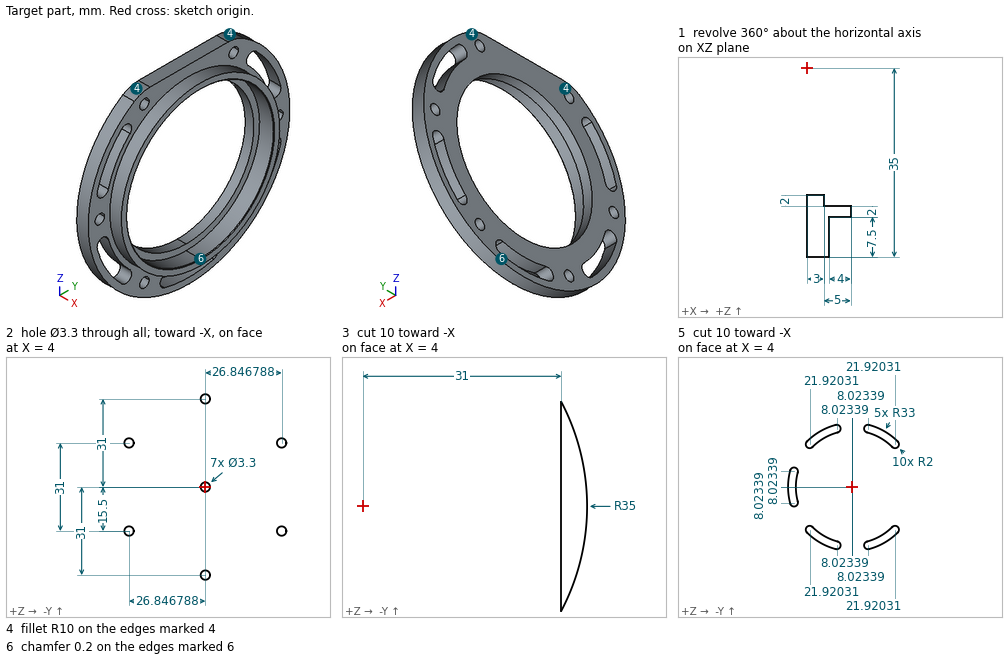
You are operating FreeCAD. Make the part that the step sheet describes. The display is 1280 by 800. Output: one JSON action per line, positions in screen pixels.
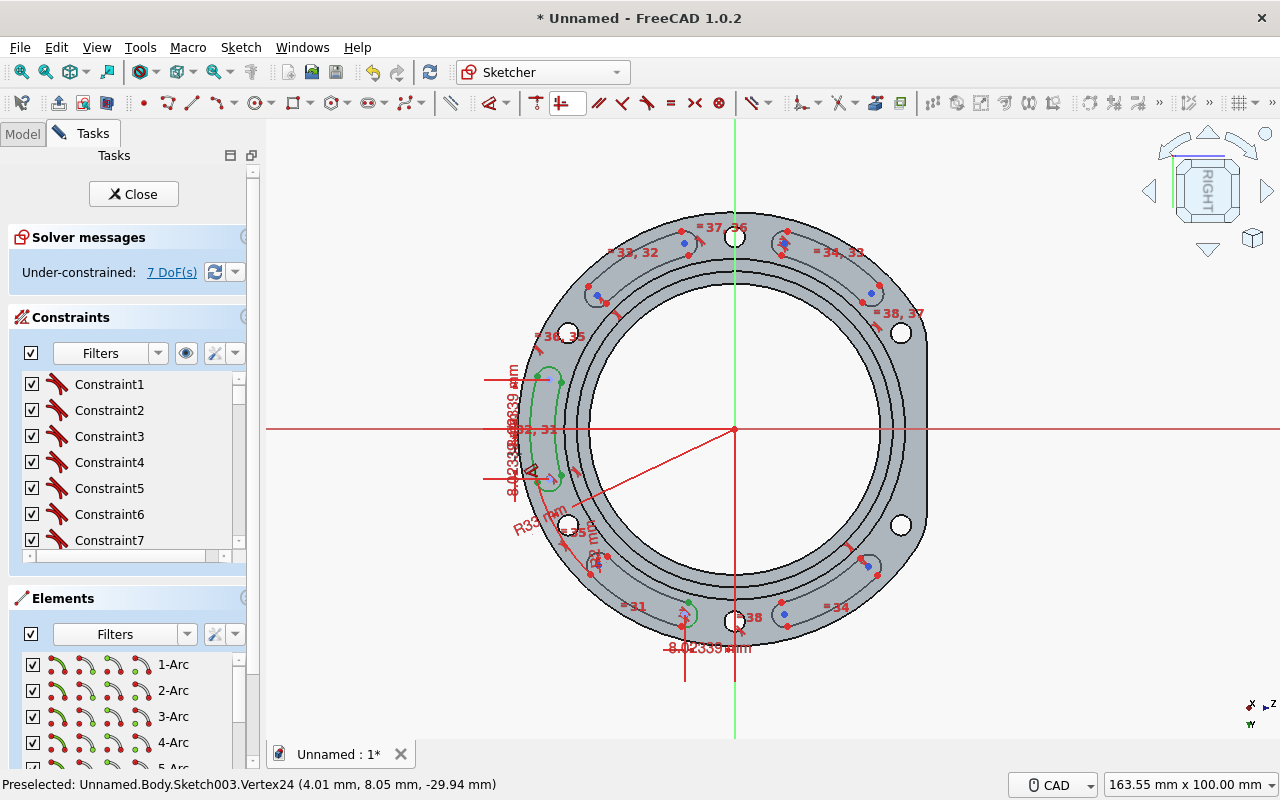
{"action": "left_click", "coordinate": [685, 244]}
{"action": "left_click", "coordinate": [710, 210]}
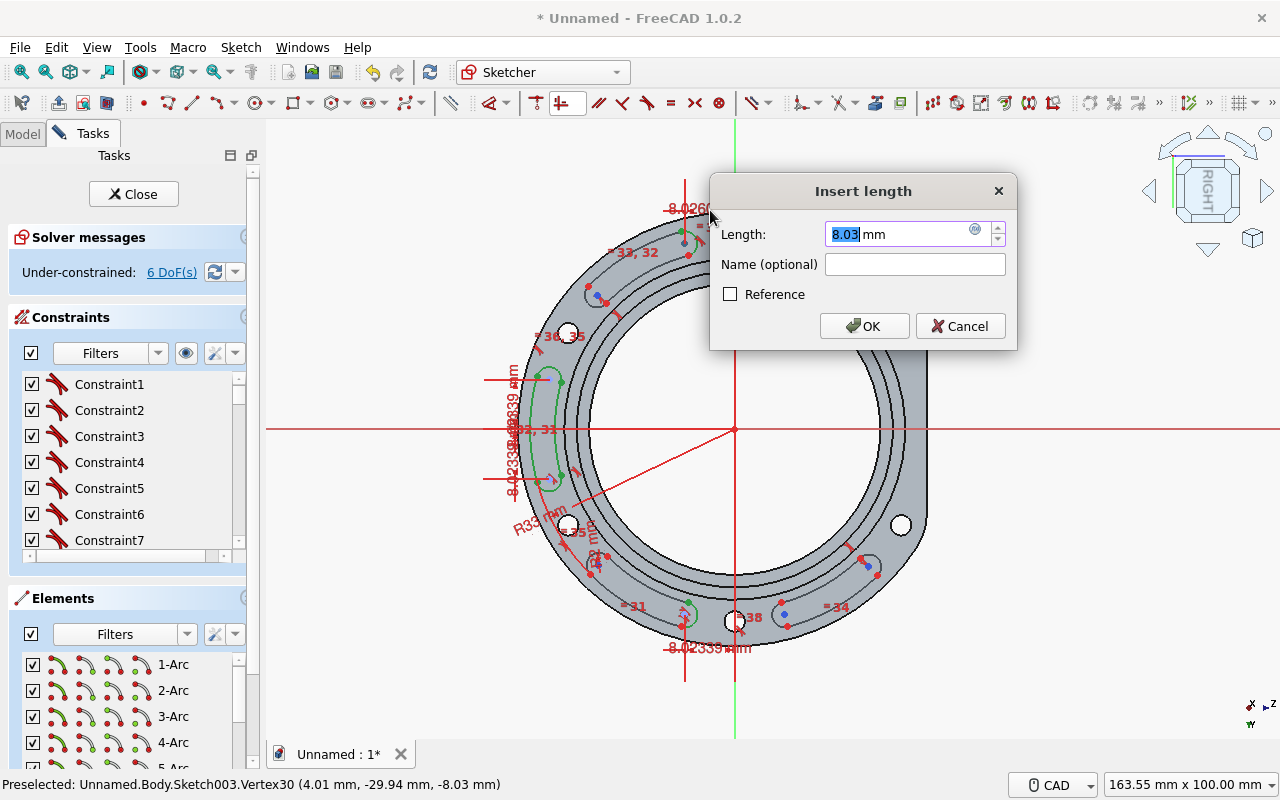
{"action": "type", "text": "8.02339"}
{"action": "key", "text": "Return"}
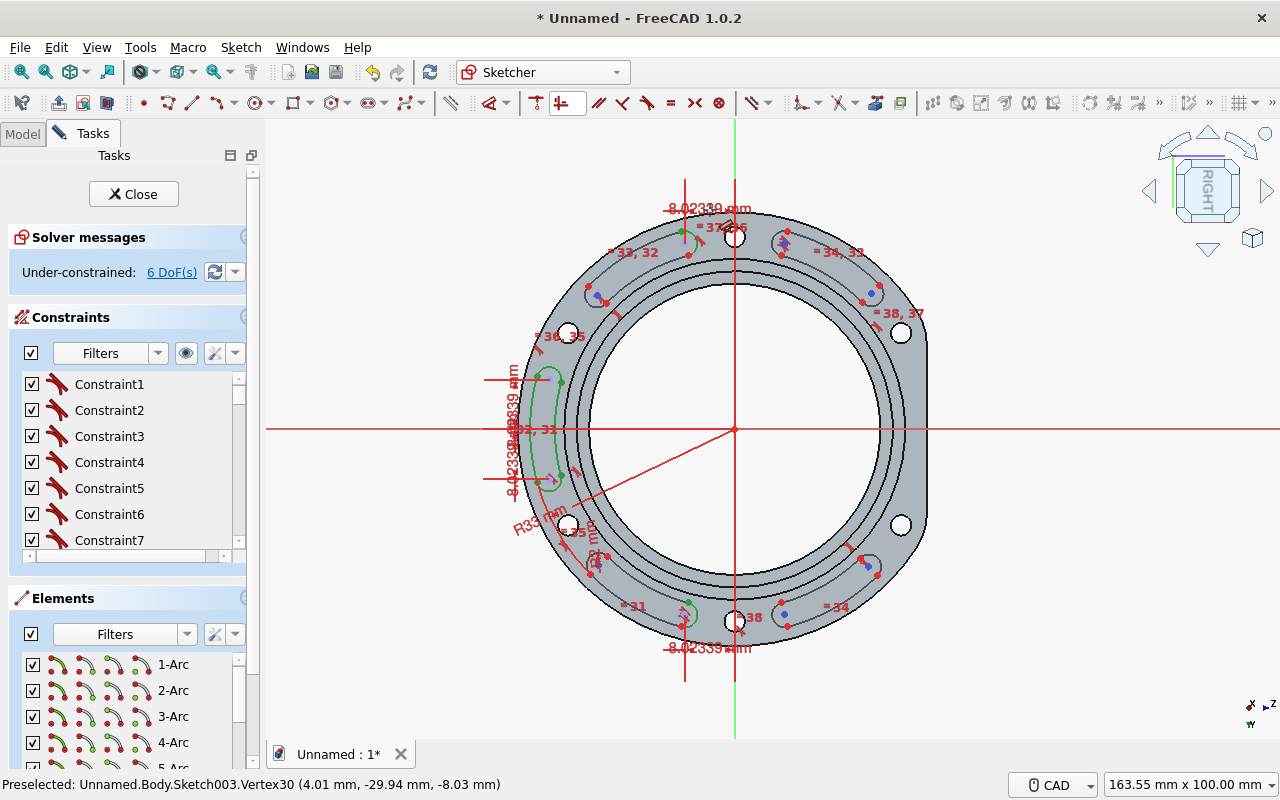
{"action": "left_click", "coordinate": [784, 244]}
{"action": "left_click", "coordinate": [759, 463]}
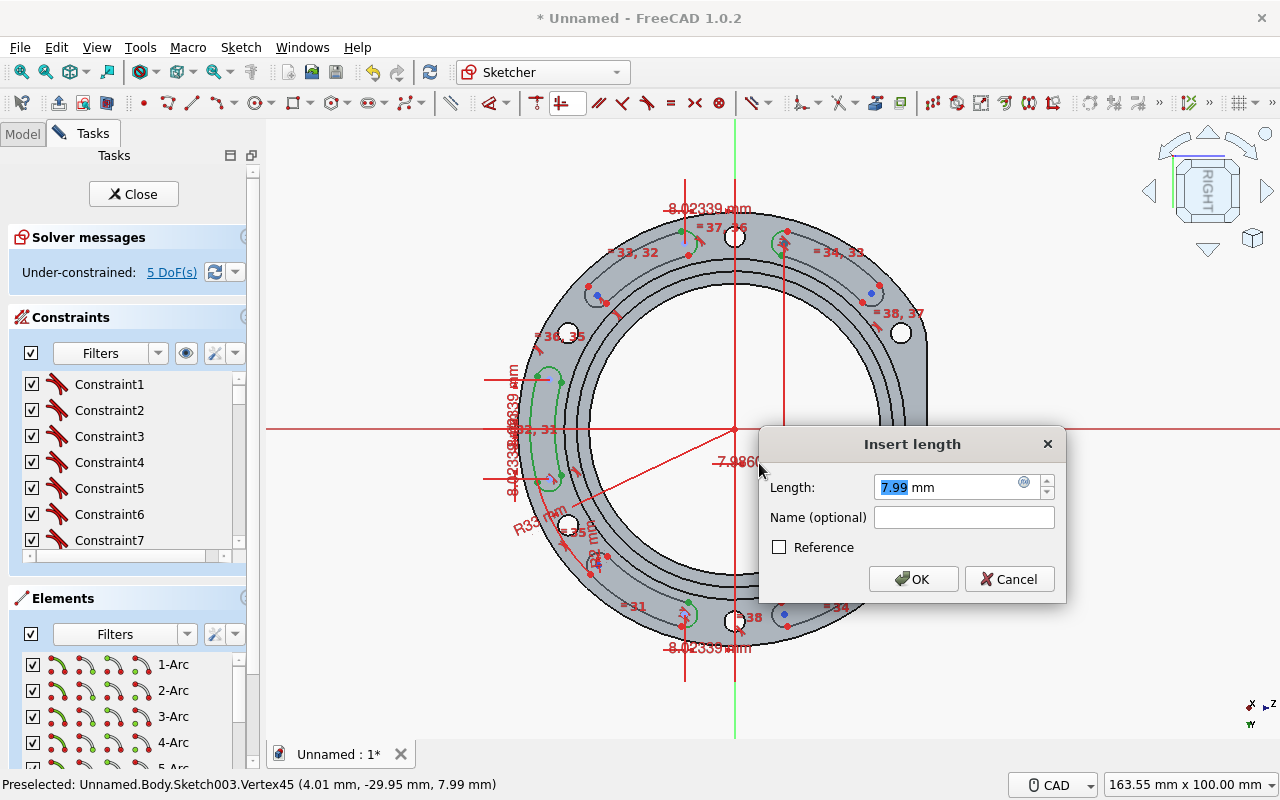
{"action": "type", "text": "8.02339"}
{"action": "key", "text": "Return"}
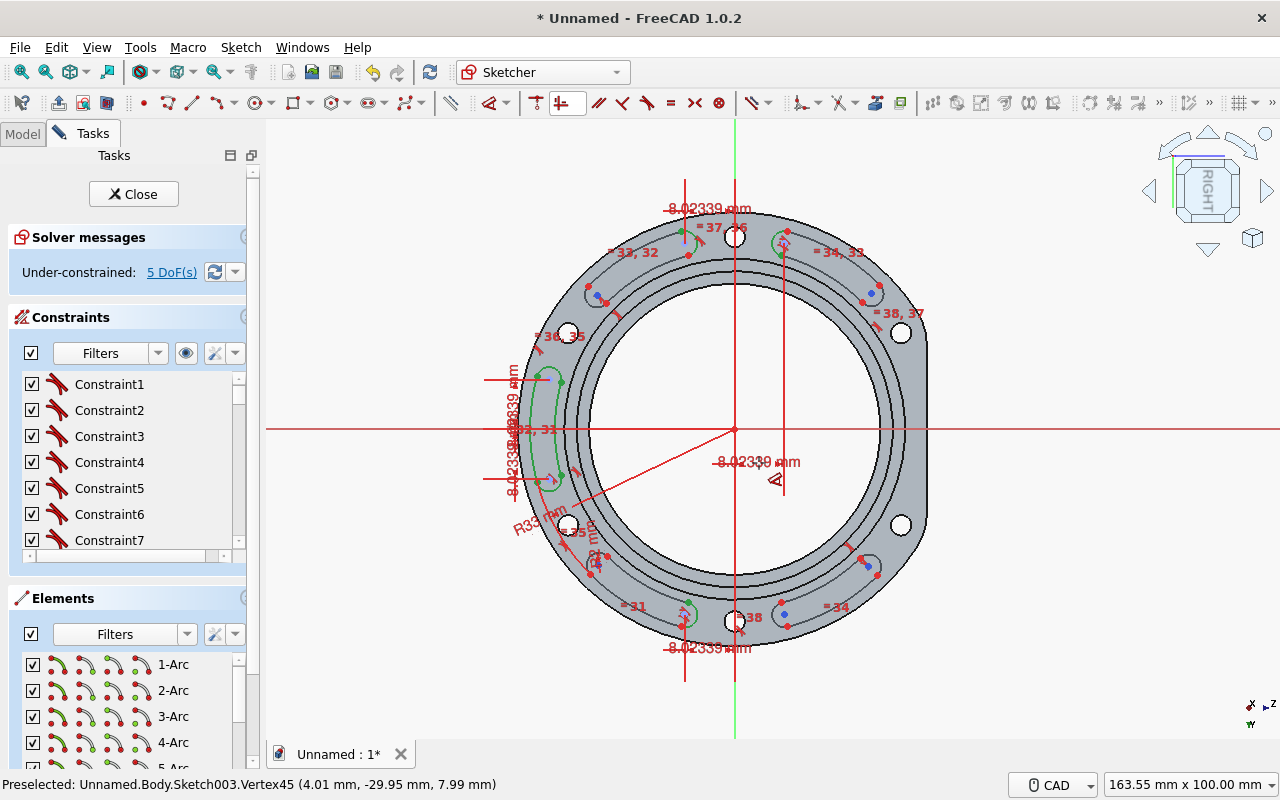
{"action": "left_click", "coordinate": [785, 615]}
{"action": "left_click", "coordinate": [760, 395]}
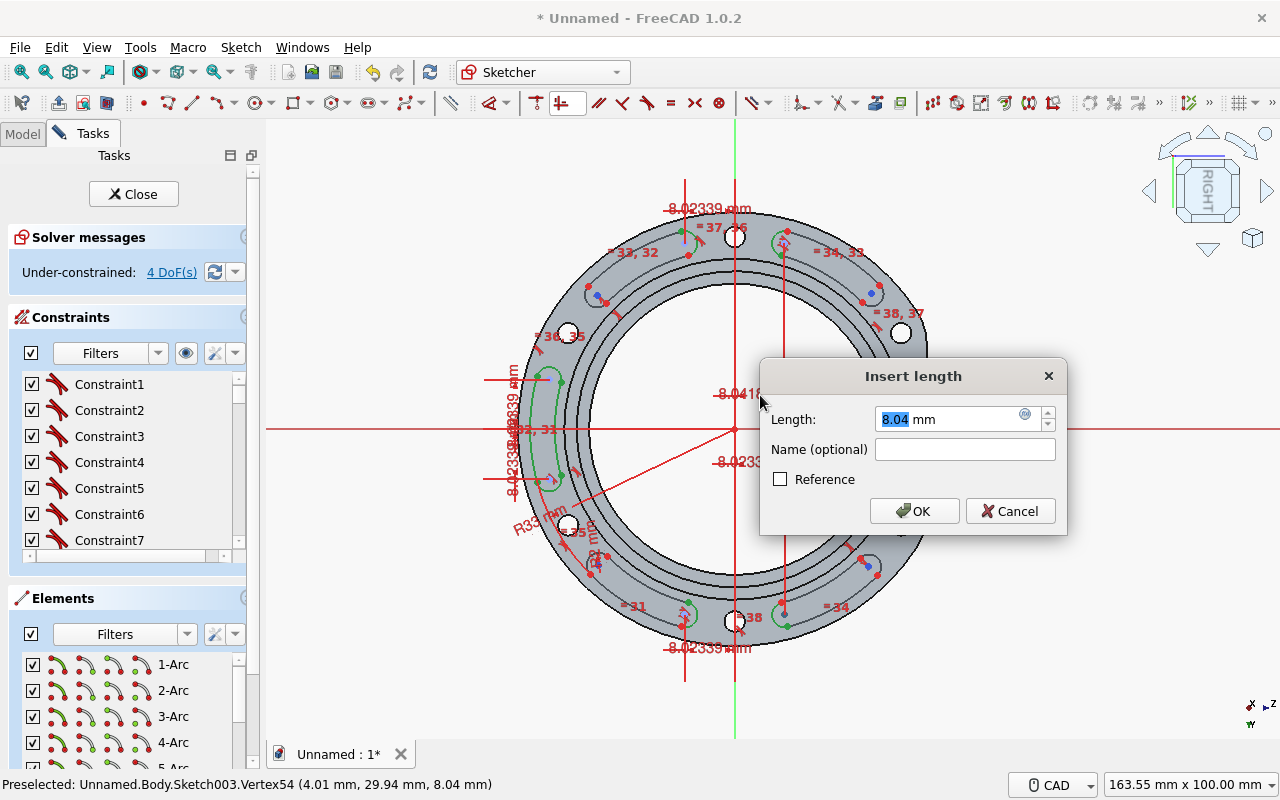
{"action": "type", "text": "8.02339"}
{"action": "key", "text": "Return"}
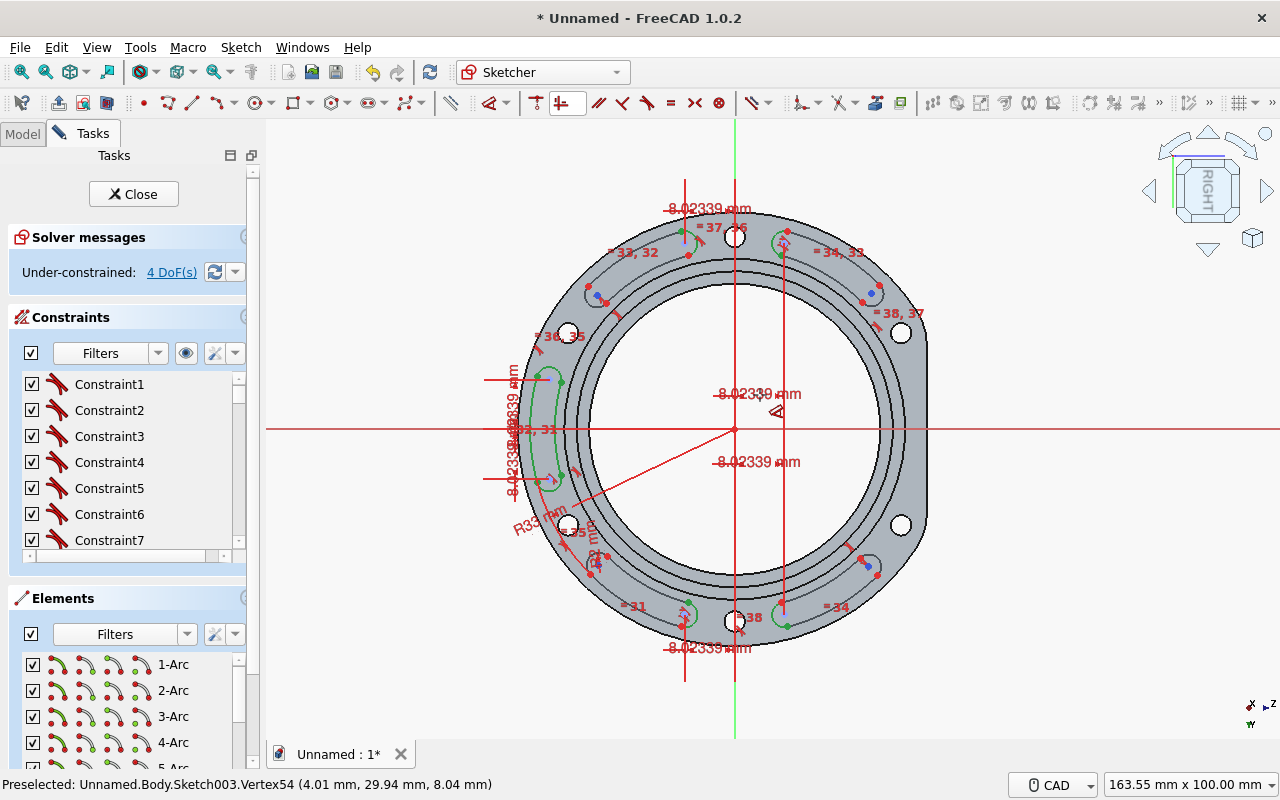
{"action": "left_click", "coordinate": [599, 565]}
{"action": "left_click", "coordinate": [714, 599]}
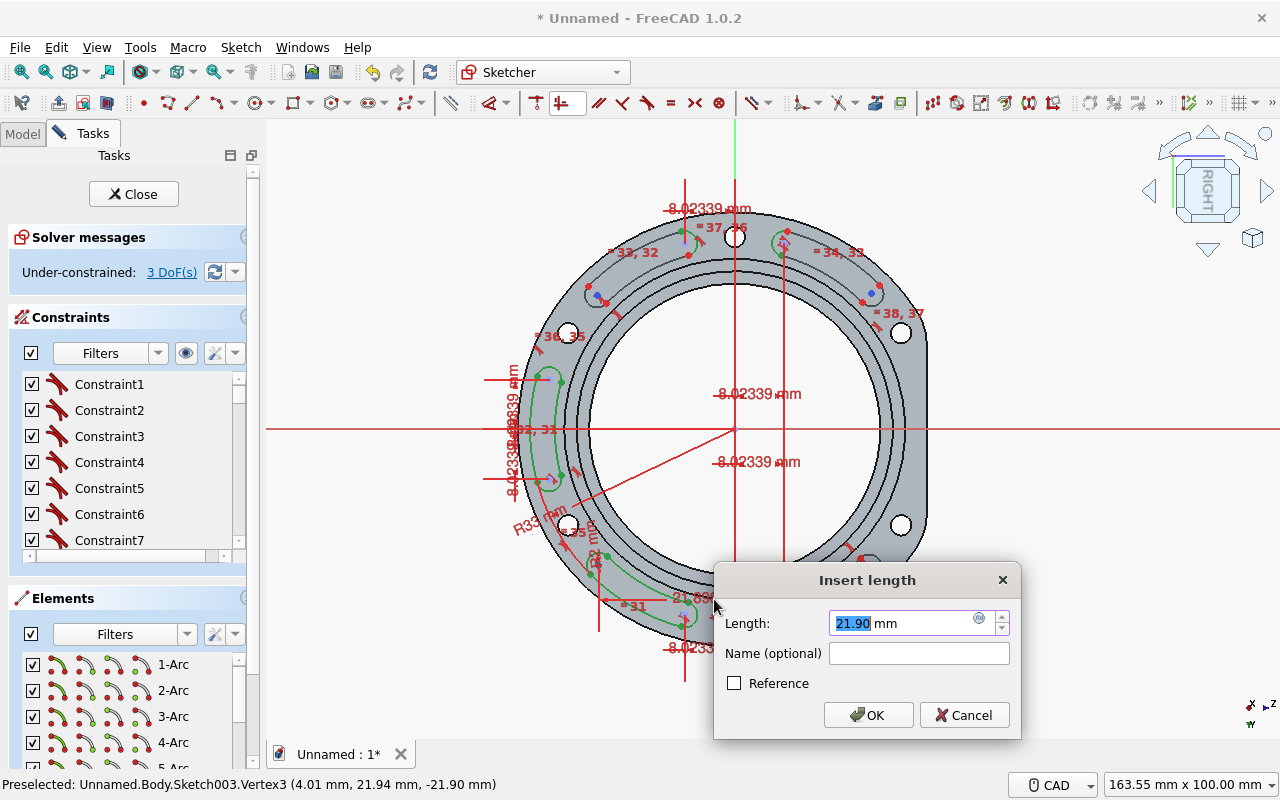
{"action": "type", "text": "21.92031"}
{"action": "key", "text": "Return"}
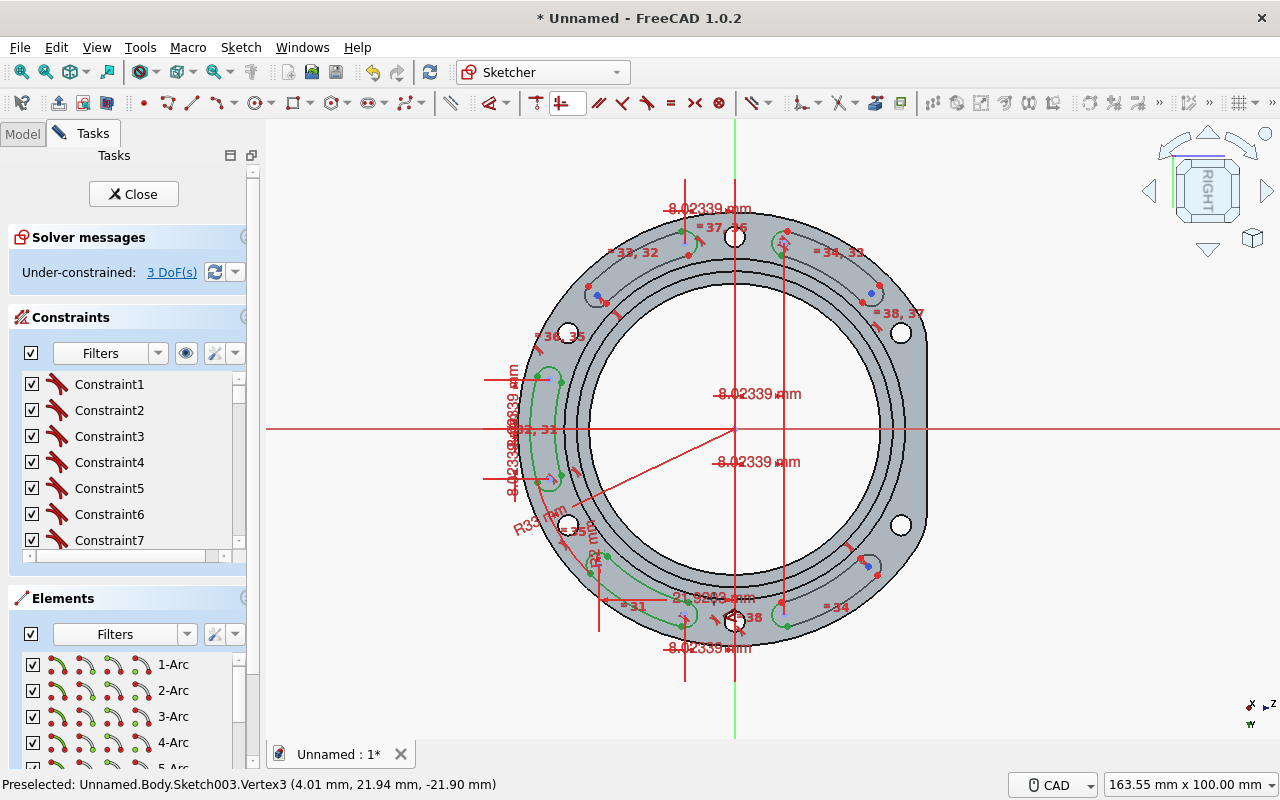
{"action": "left_click", "coordinate": [597, 295]}
{"action": "left_click", "coordinate": [714, 261]}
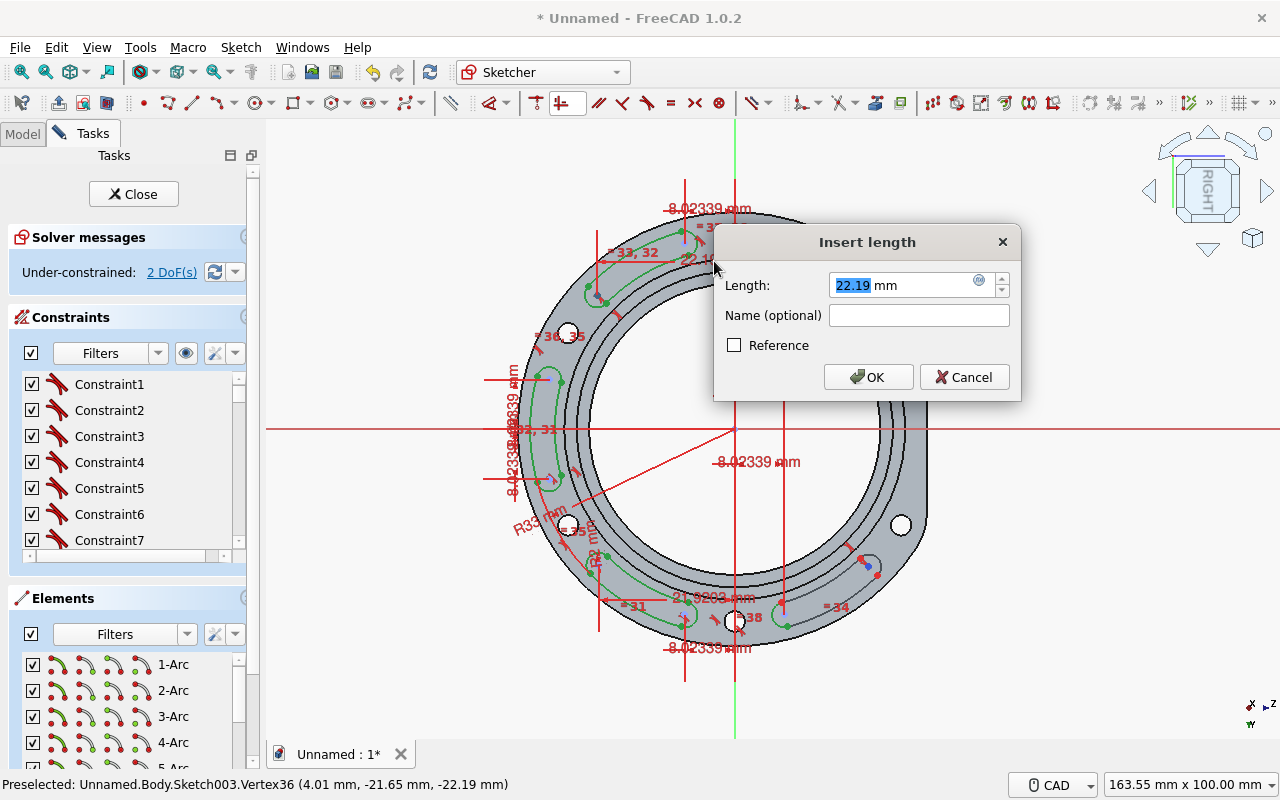
{"action": "type", "text": "21.92031"}
{"action": "key", "text": "Return"}